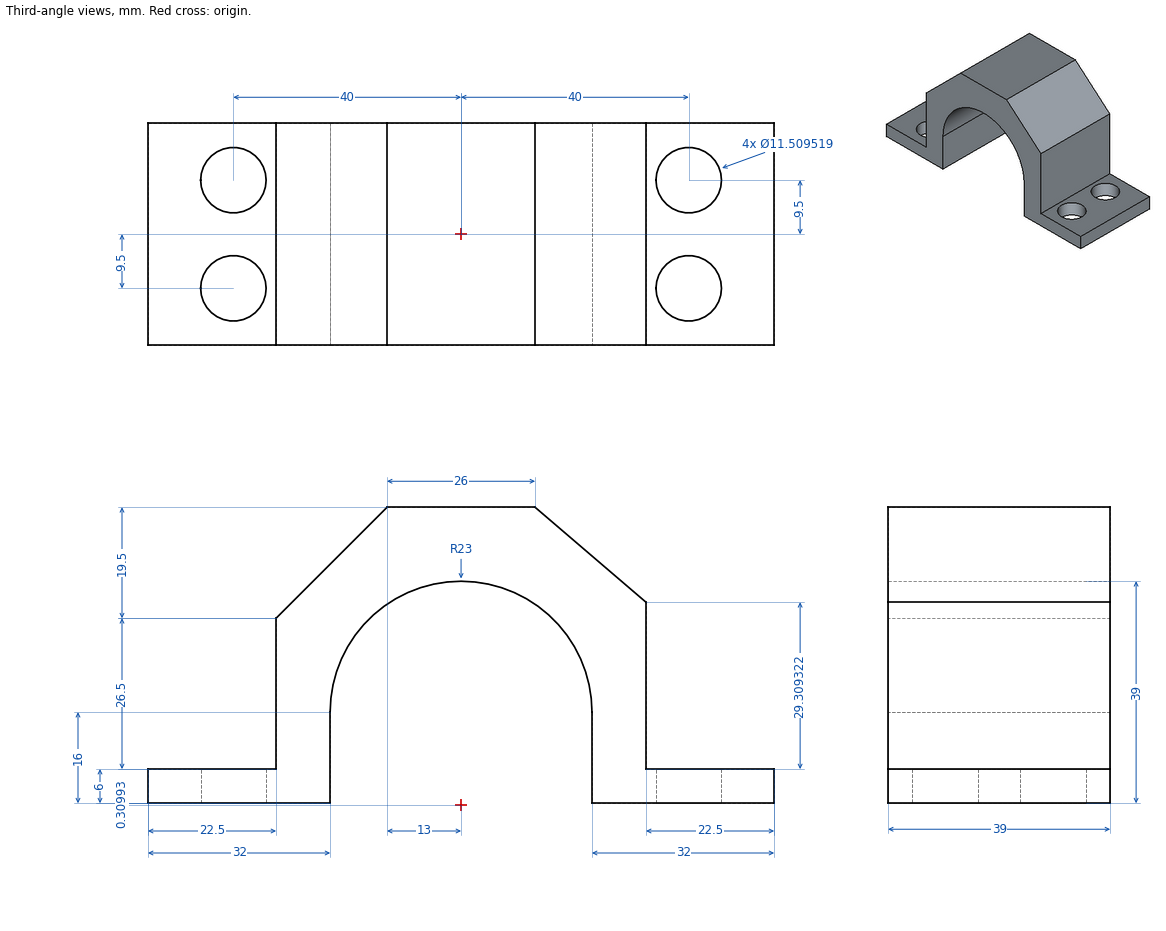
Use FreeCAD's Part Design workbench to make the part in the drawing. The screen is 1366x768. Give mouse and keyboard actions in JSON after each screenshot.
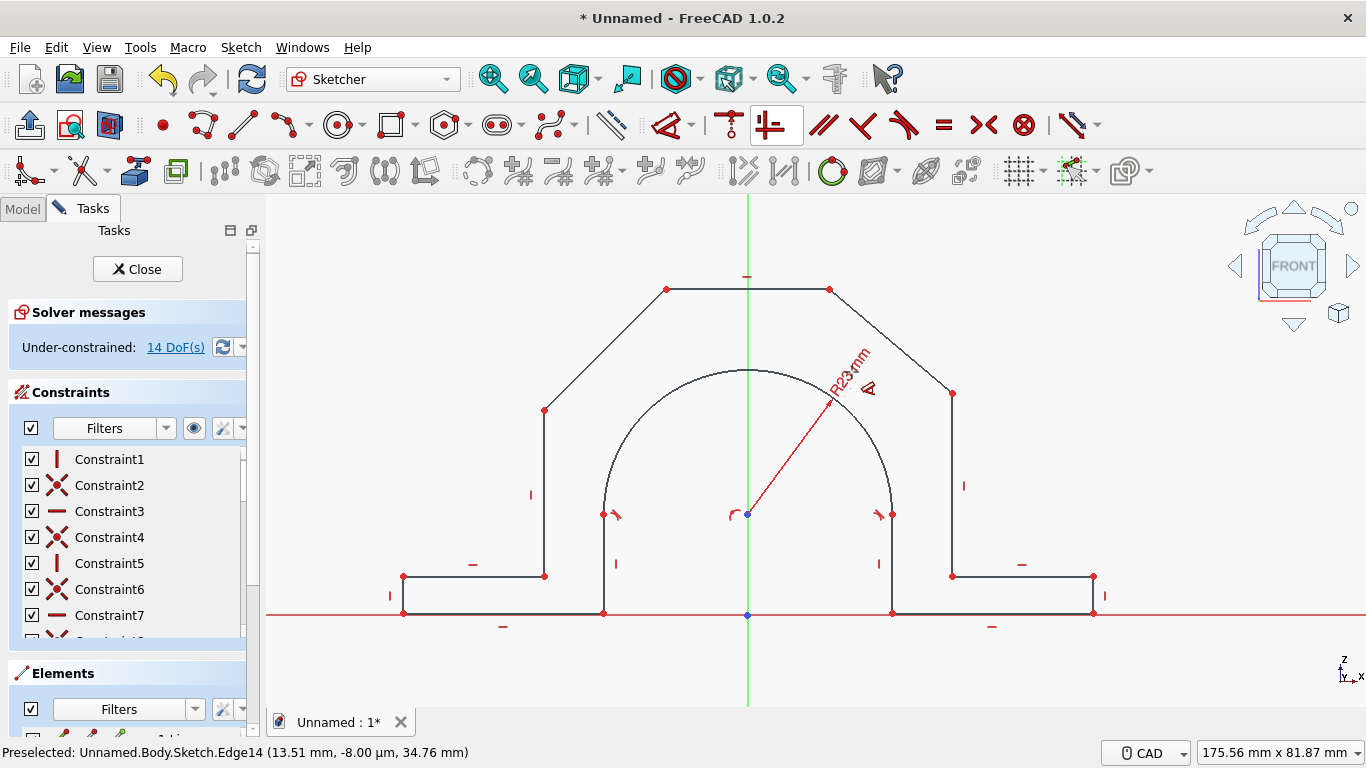
{"action": "scroll", "coordinate": [403, 603], "scroll_direction": "up", "scroll_amount": 2}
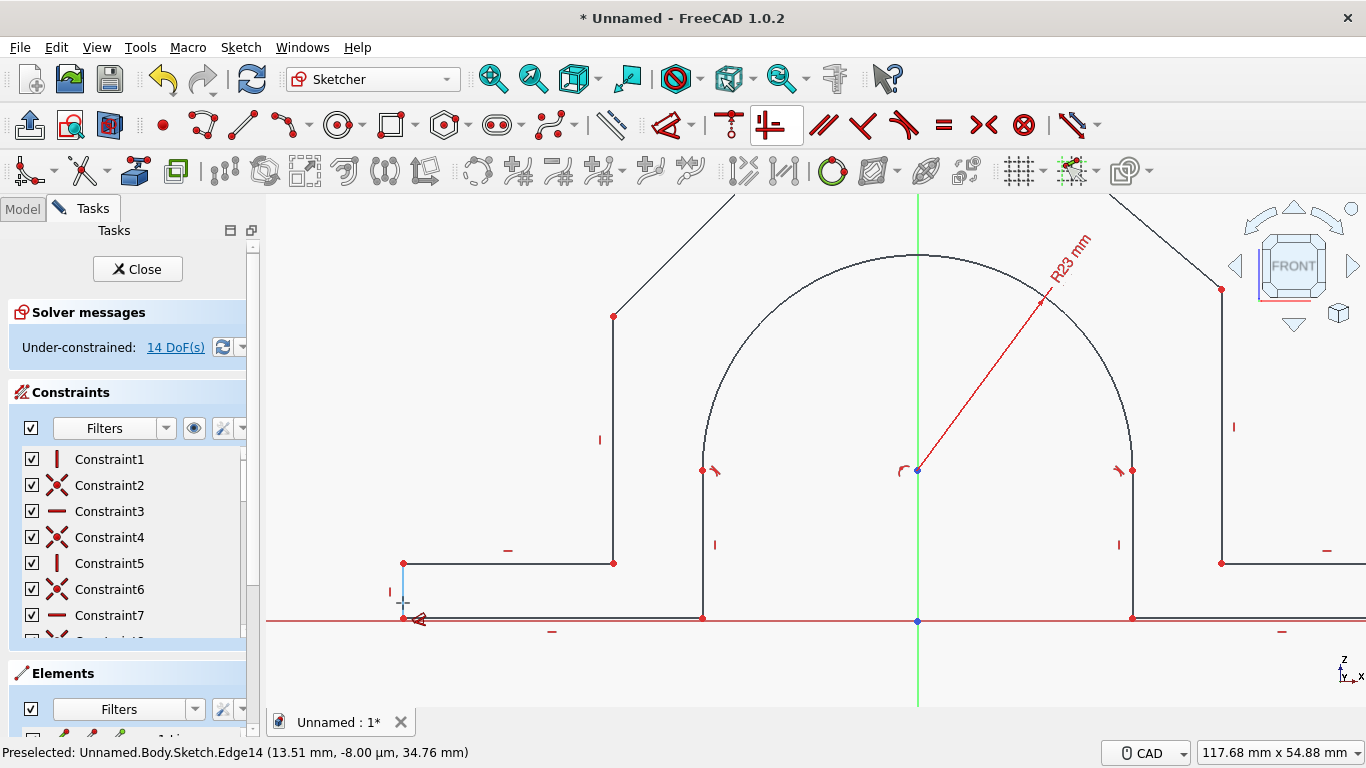
{"action": "left_click", "coordinate": [403, 602]}
{"action": "left_click", "coordinate": [369, 591]}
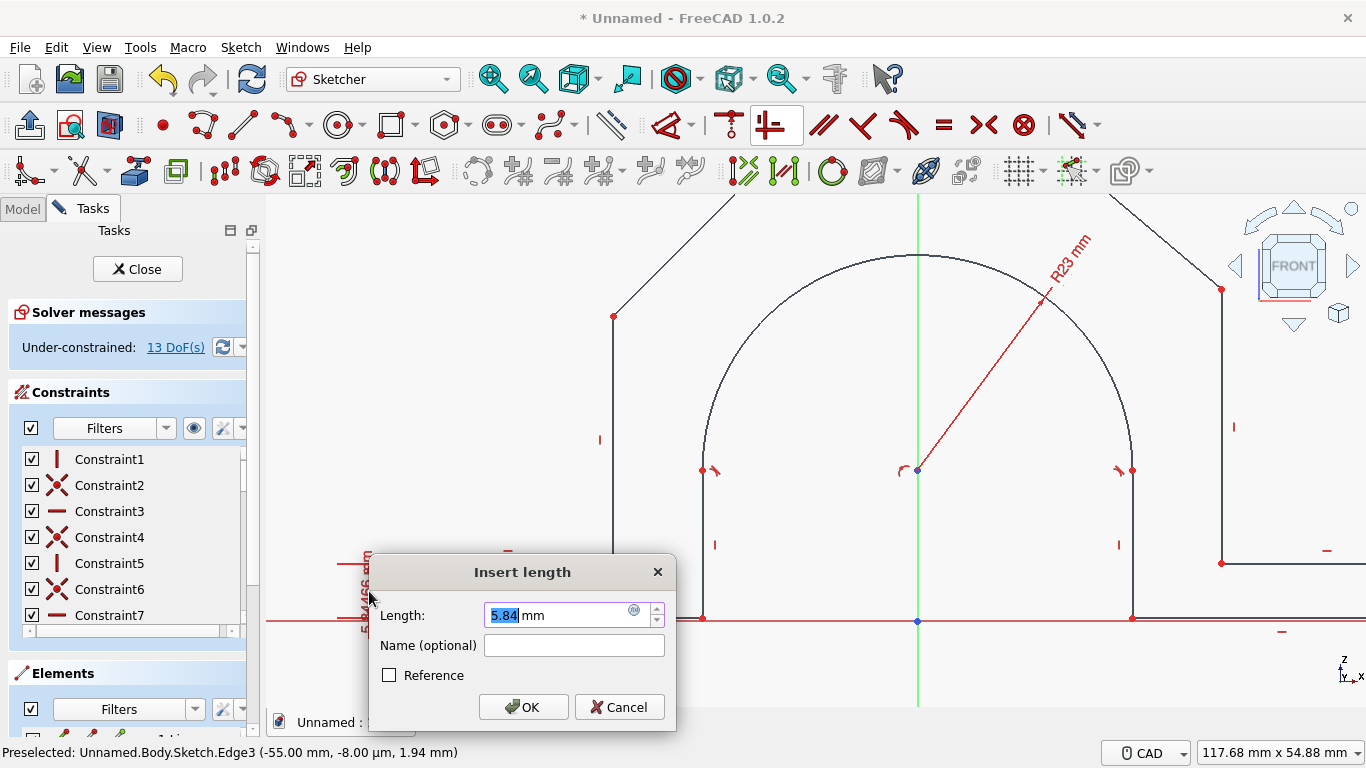
{"action": "type", "text": "6"}
{"action": "key", "text": "Return"}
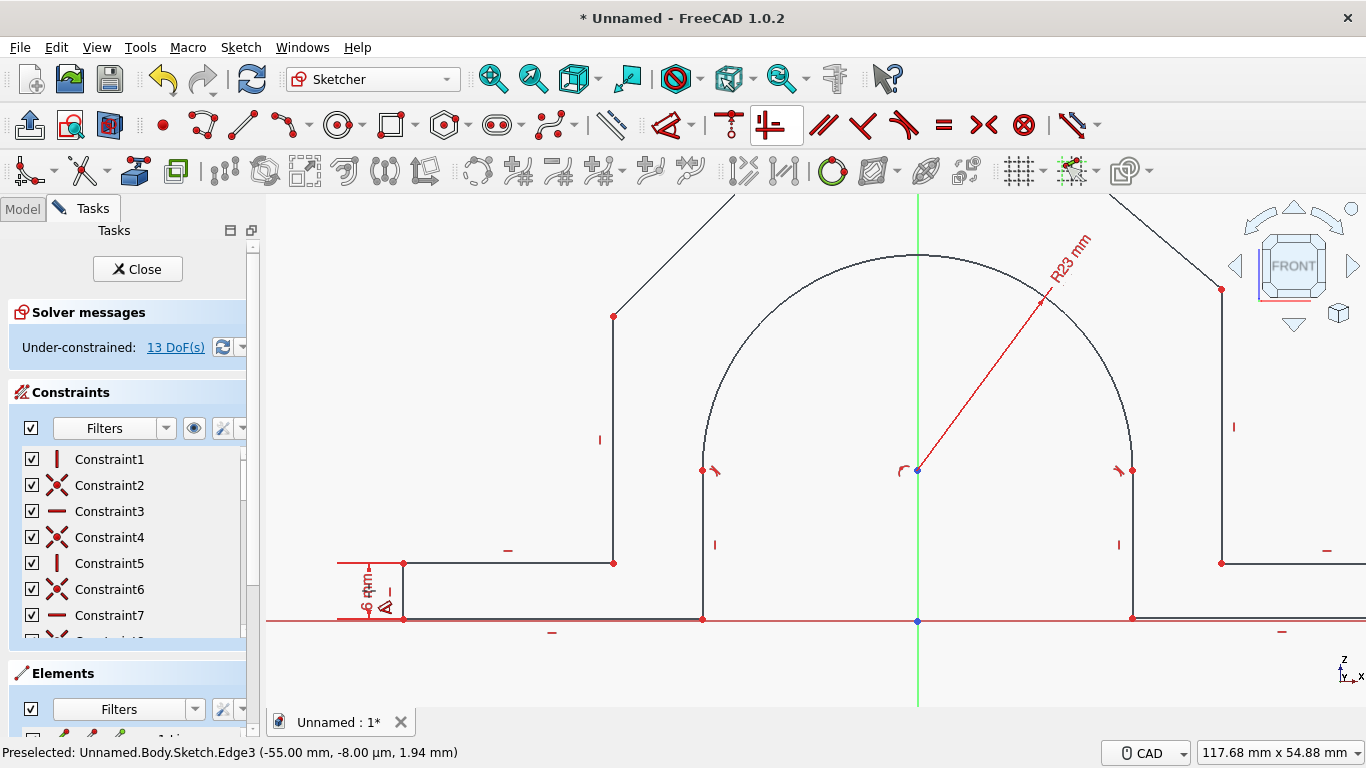
{"action": "scroll", "coordinate": [402, 601], "scroll_direction": "down", "scroll_amount": 2}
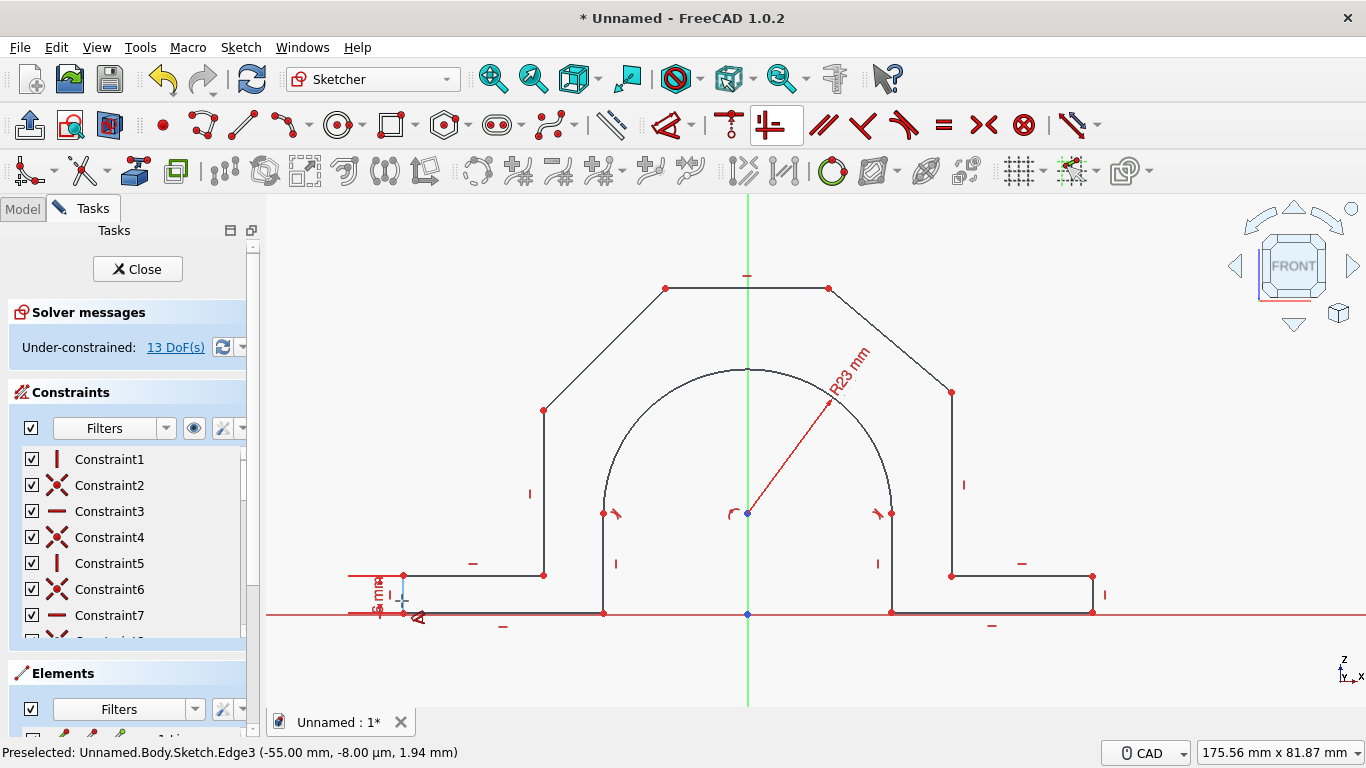
{"action": "scroll", "coordinate": [1093, 587], "scroll_direction": "up", "scroll_amount": 2}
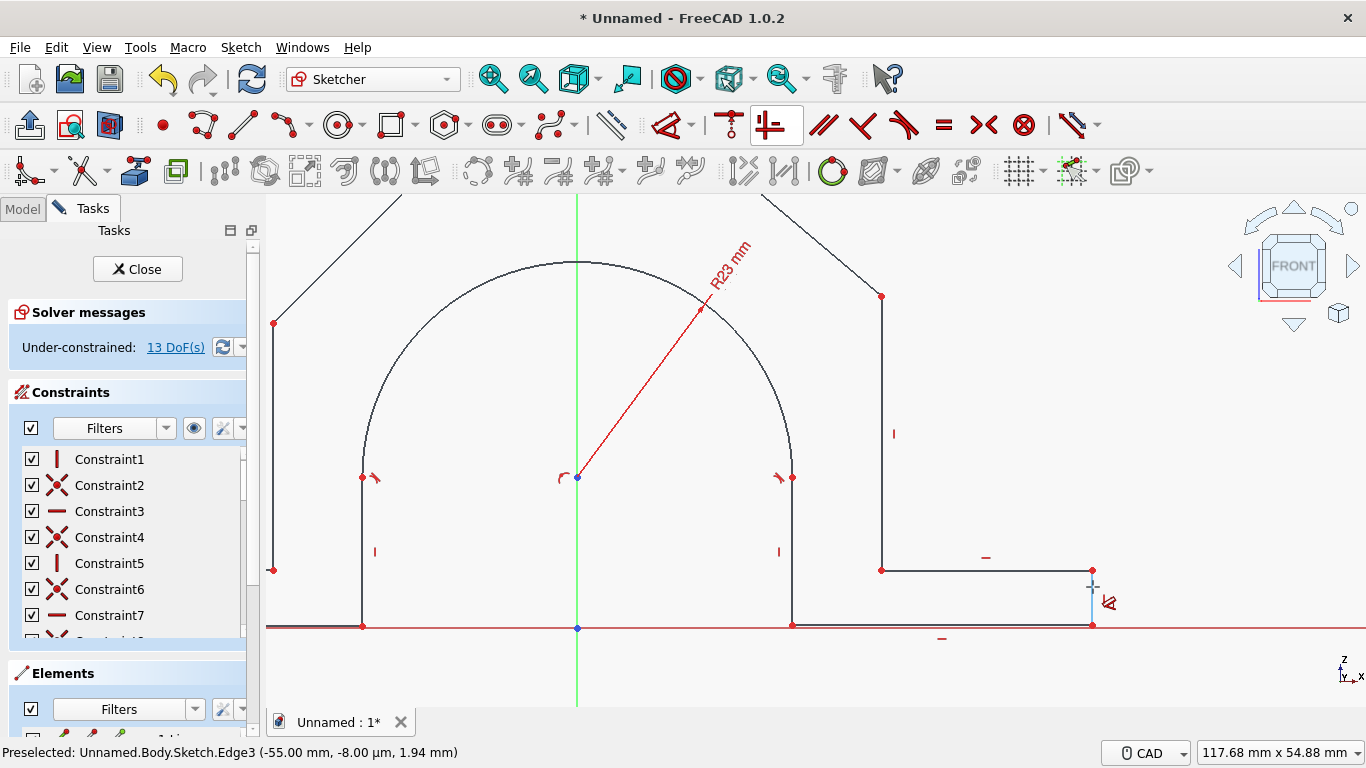
{"action": "left_click", "coordinate": [1092, 587]}
{"action": "left_click", "coordinate": [1126, 598]}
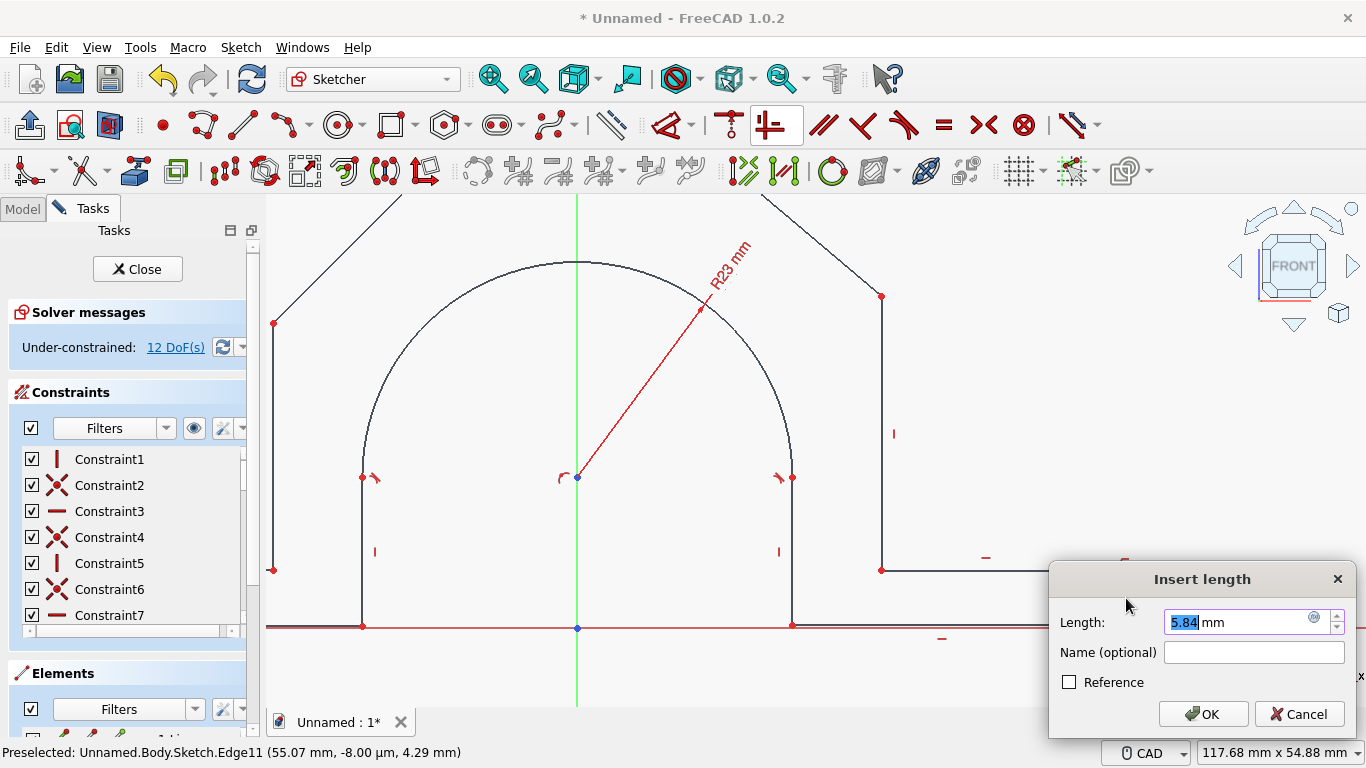
{"action": "type", "text": "6"}
{"action": "key", "text": "Return"}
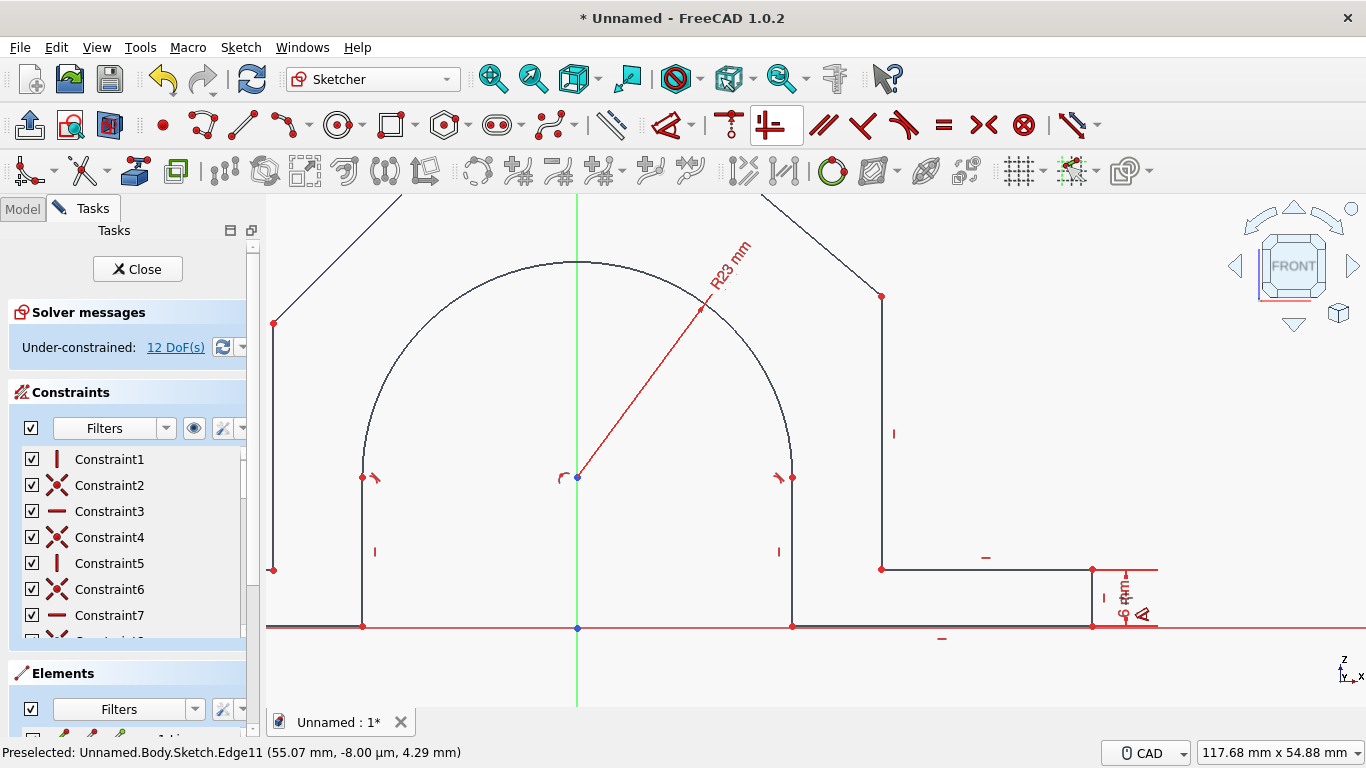
{"action": "left_click", "coordinate": [362, 522]}
{"action": "left_click", "coordinate": [328, 552]}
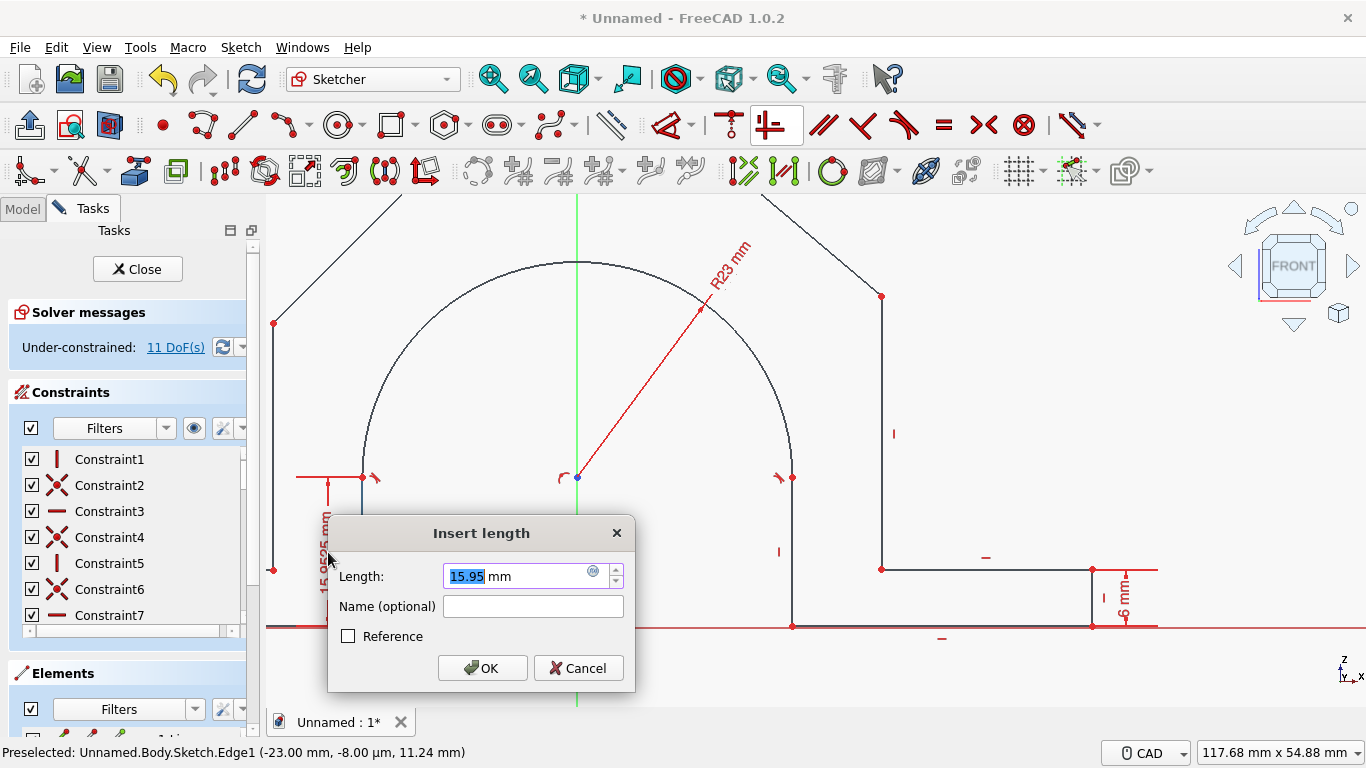
{"action": "type", "text": "16"}
{"action": "key", "text": "Return"}